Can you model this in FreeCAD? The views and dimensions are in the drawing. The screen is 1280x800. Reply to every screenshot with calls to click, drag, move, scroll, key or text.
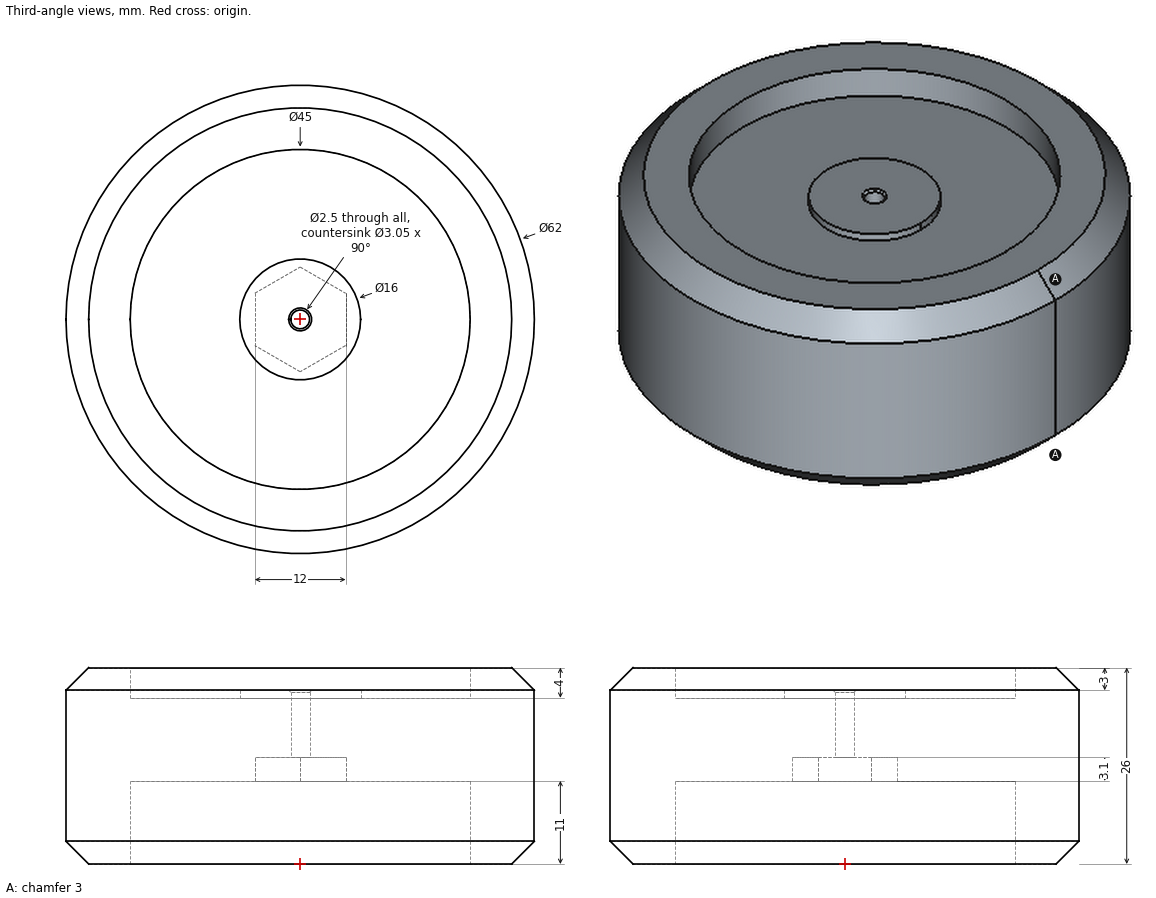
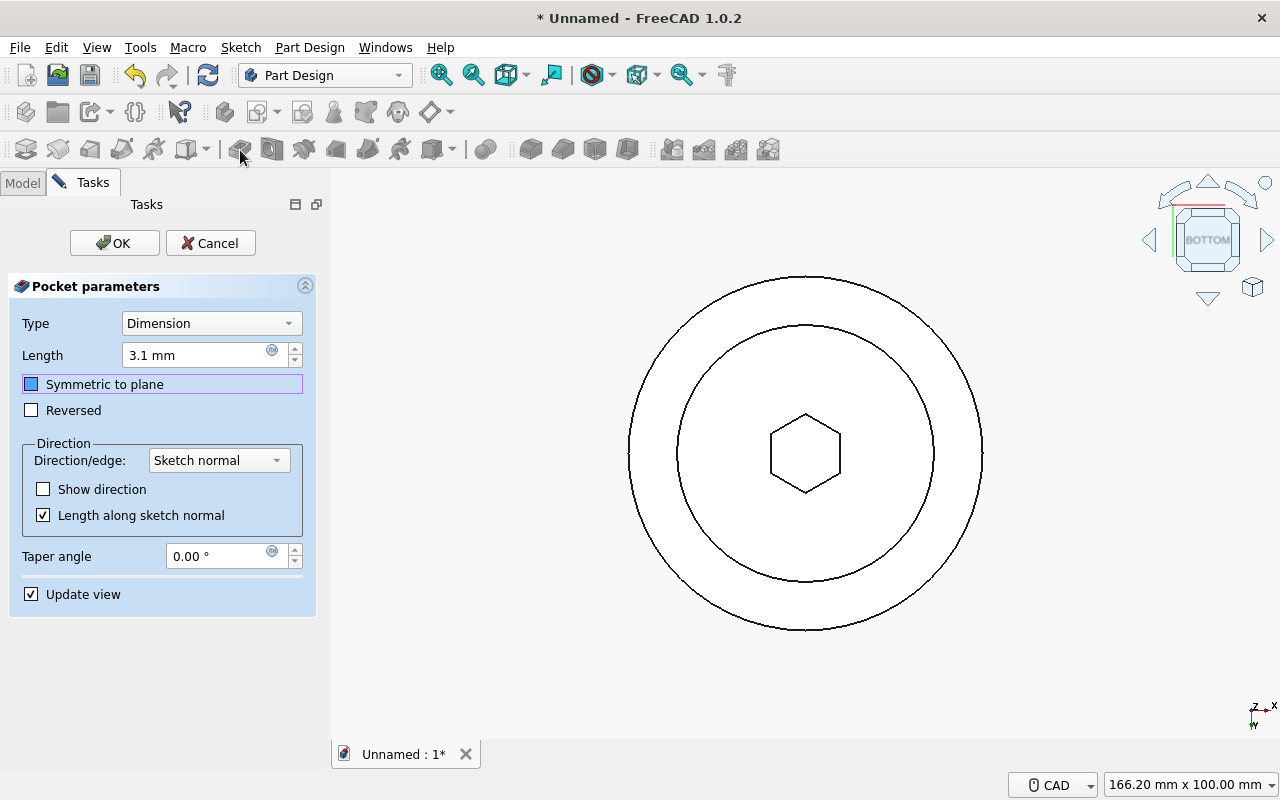
click(115, 243)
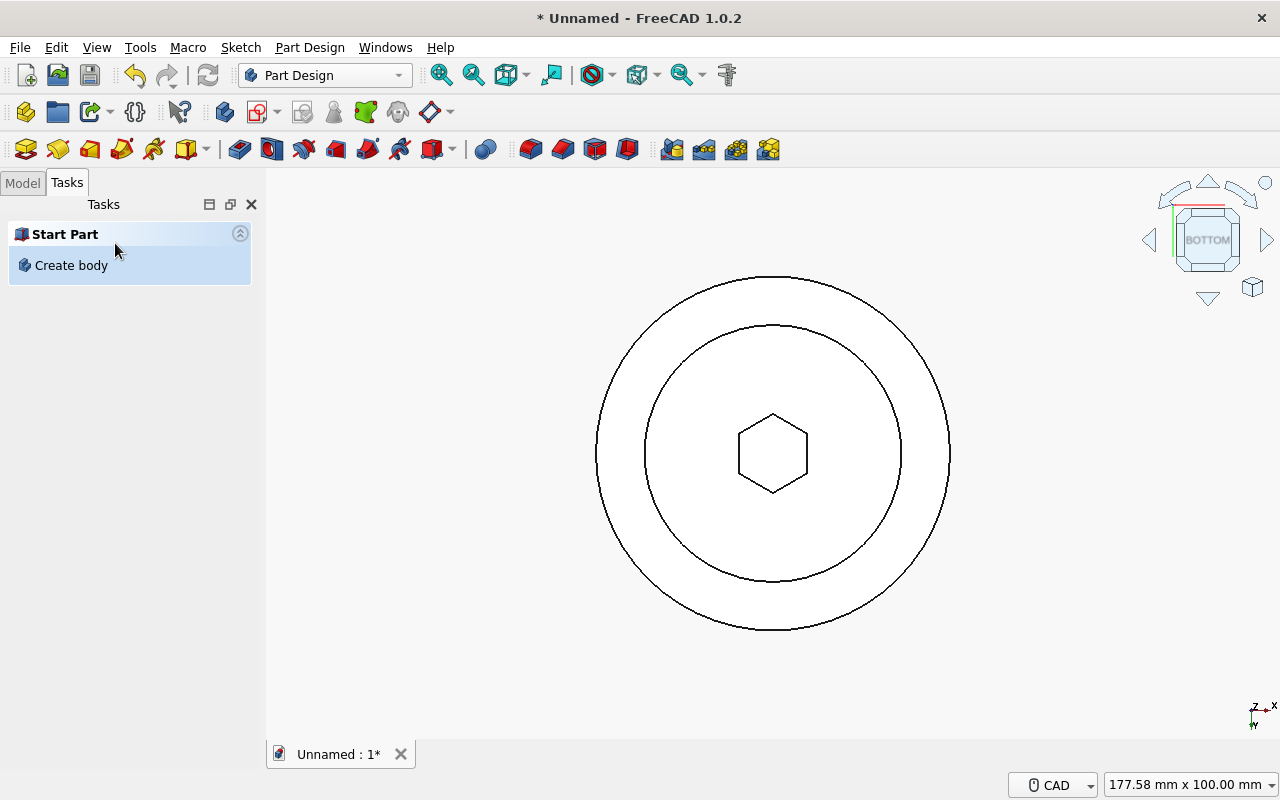
click(23, 182)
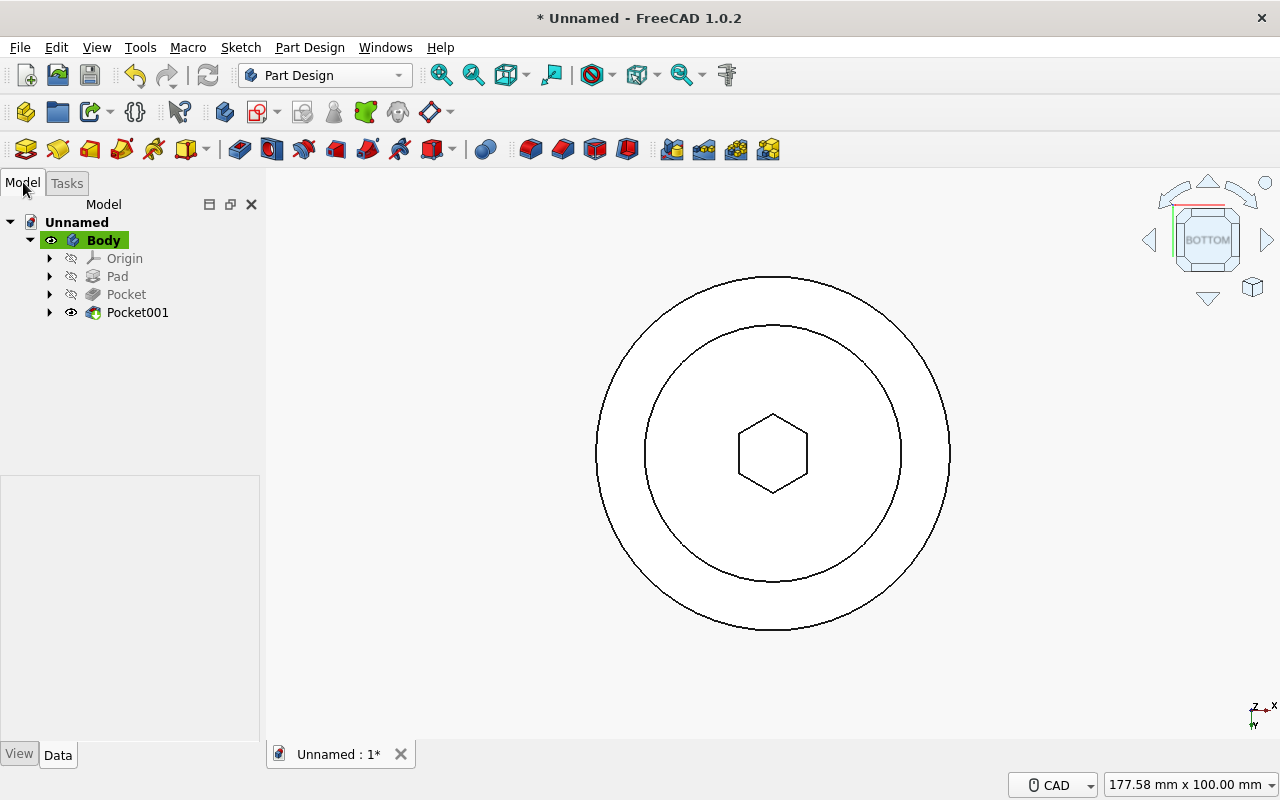
click(50, 258)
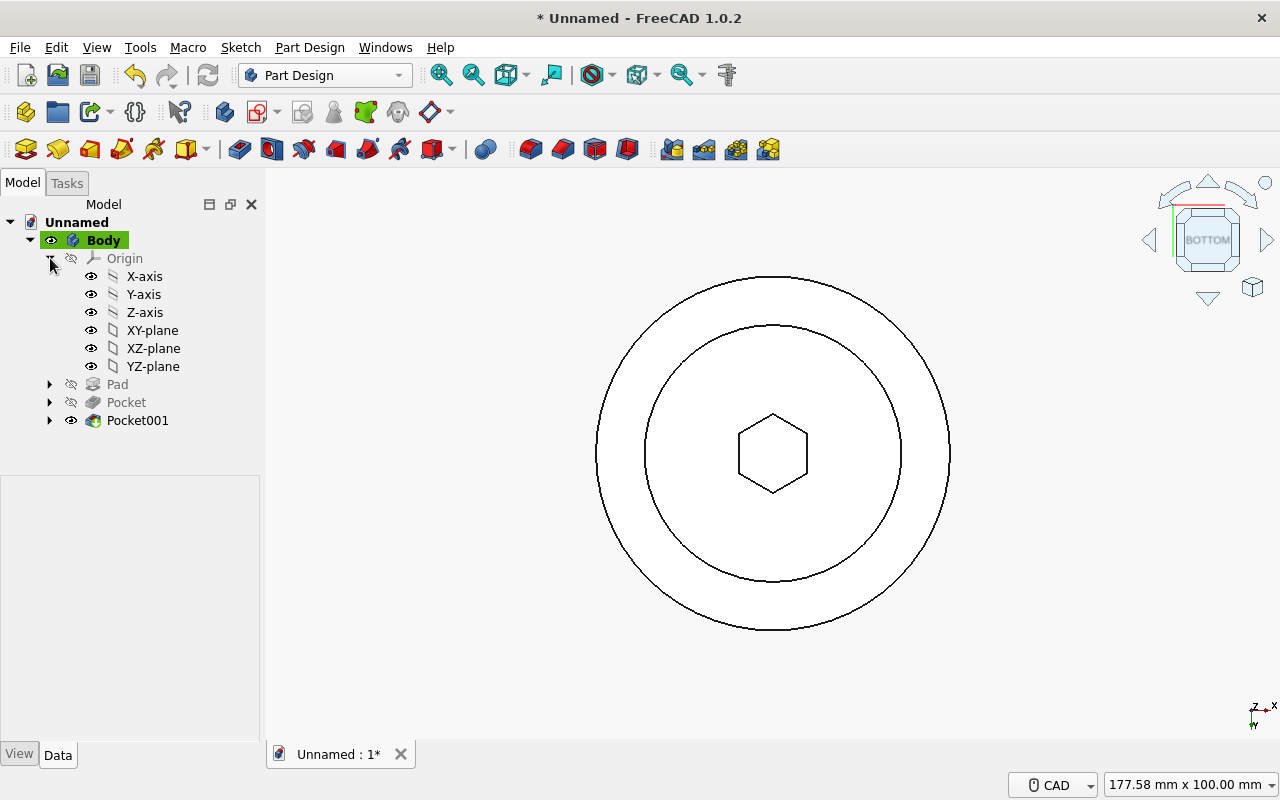
click(136, 330)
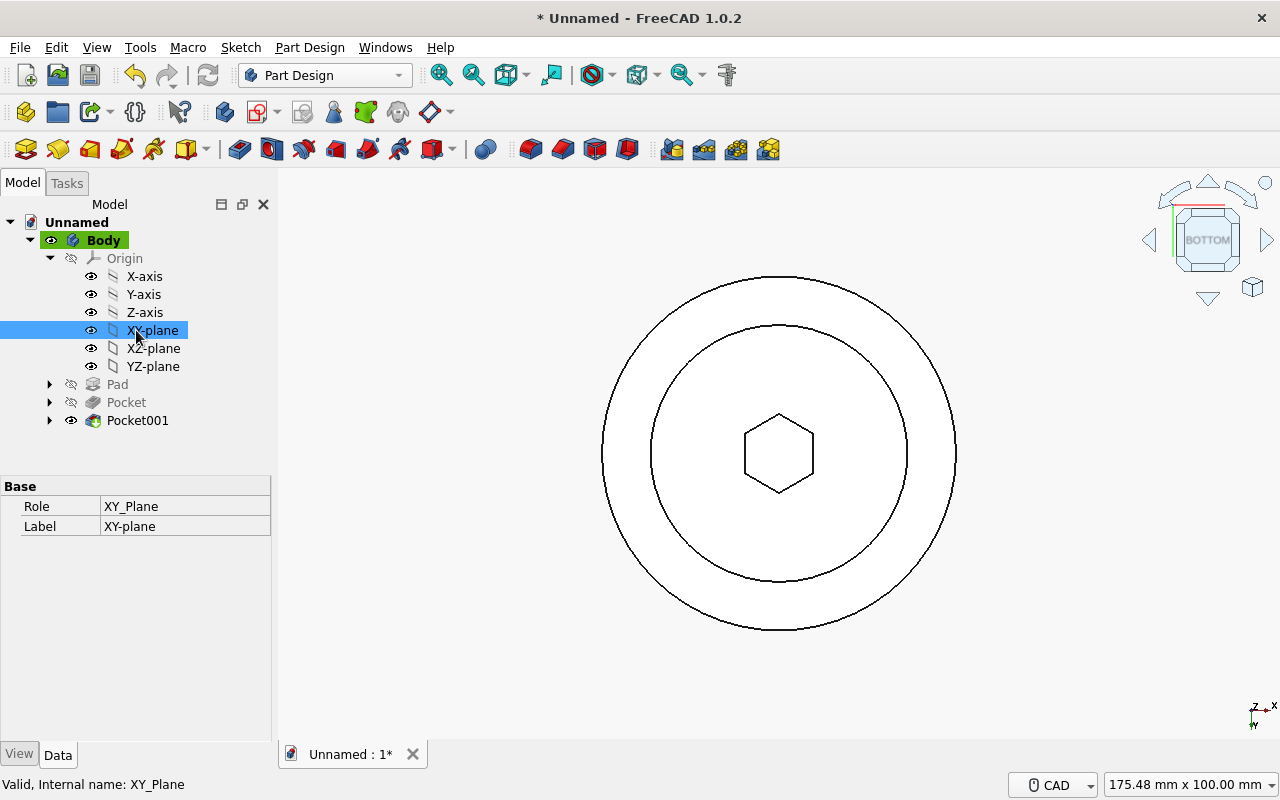
click(430, 112)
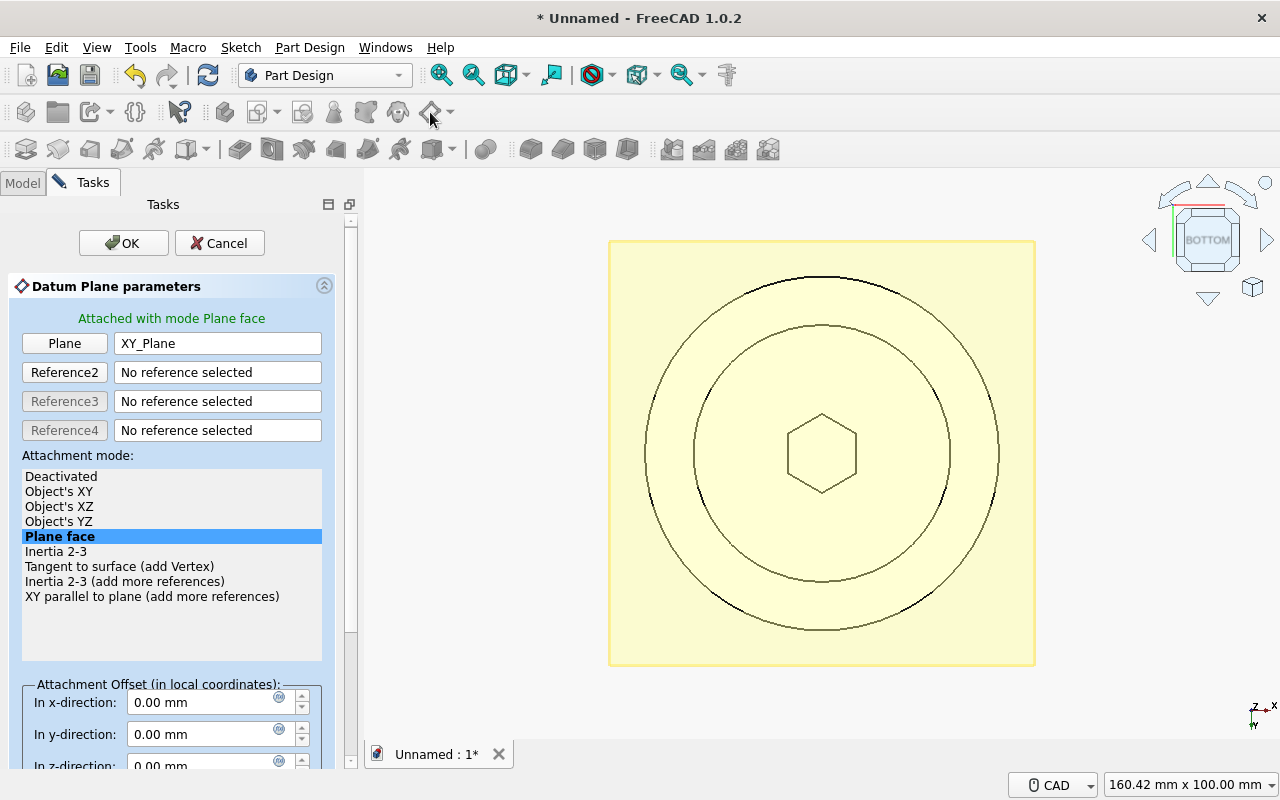
scroll(351, 491, down, 2)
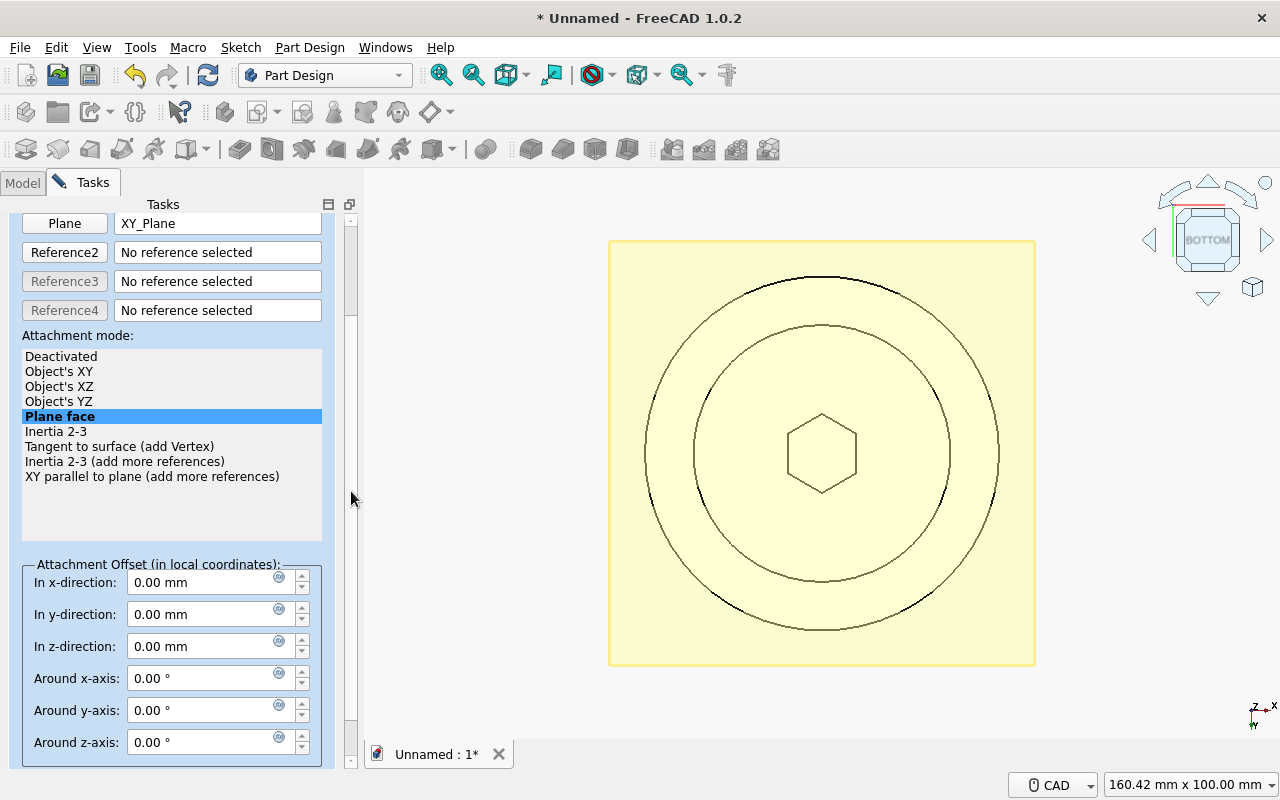
triple_click(210, 646)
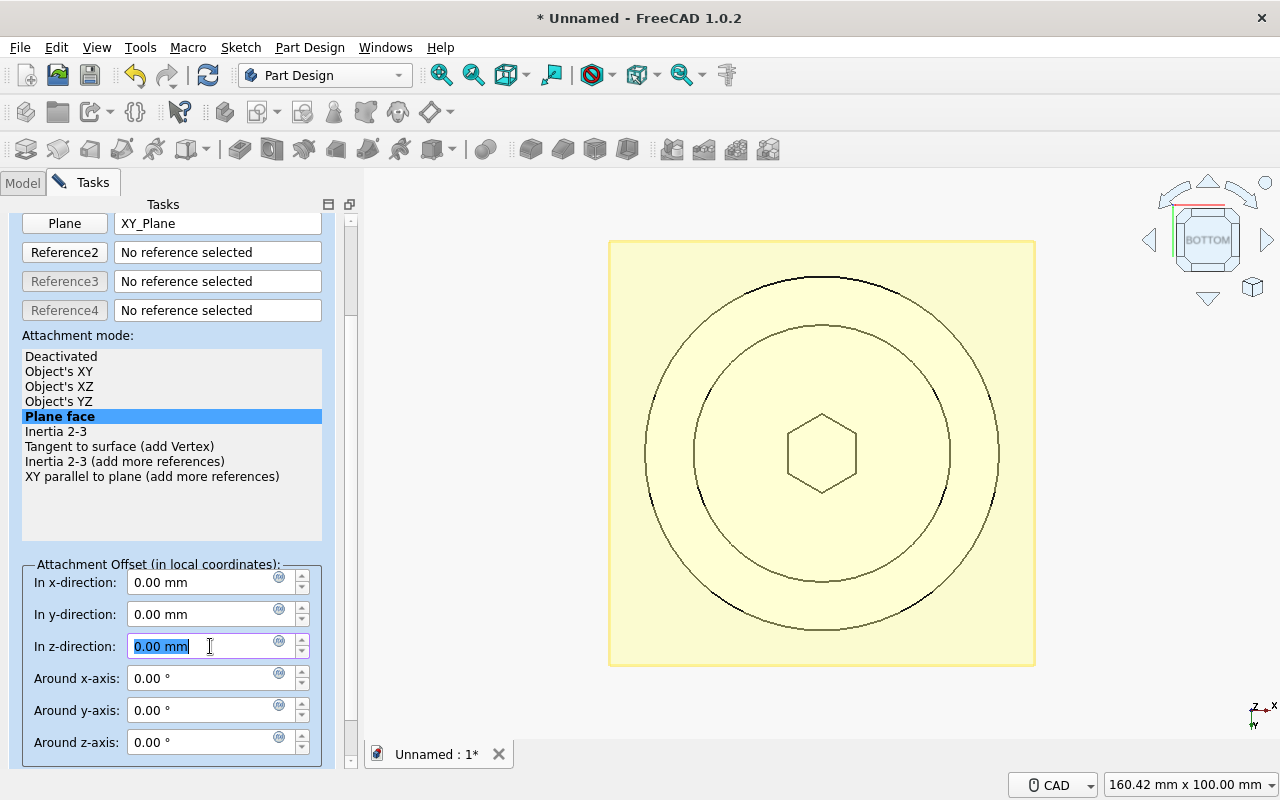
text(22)
key(Tab)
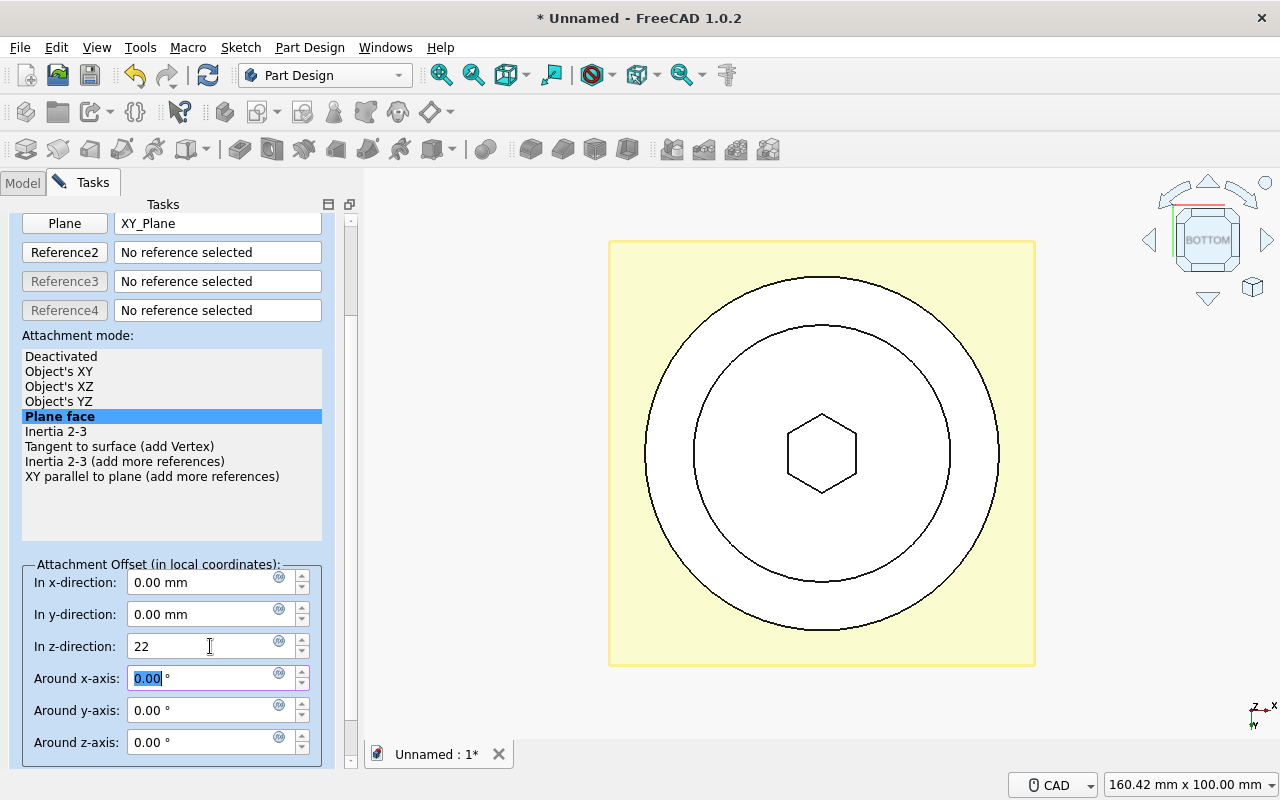
scroll(351, 491, up, 3)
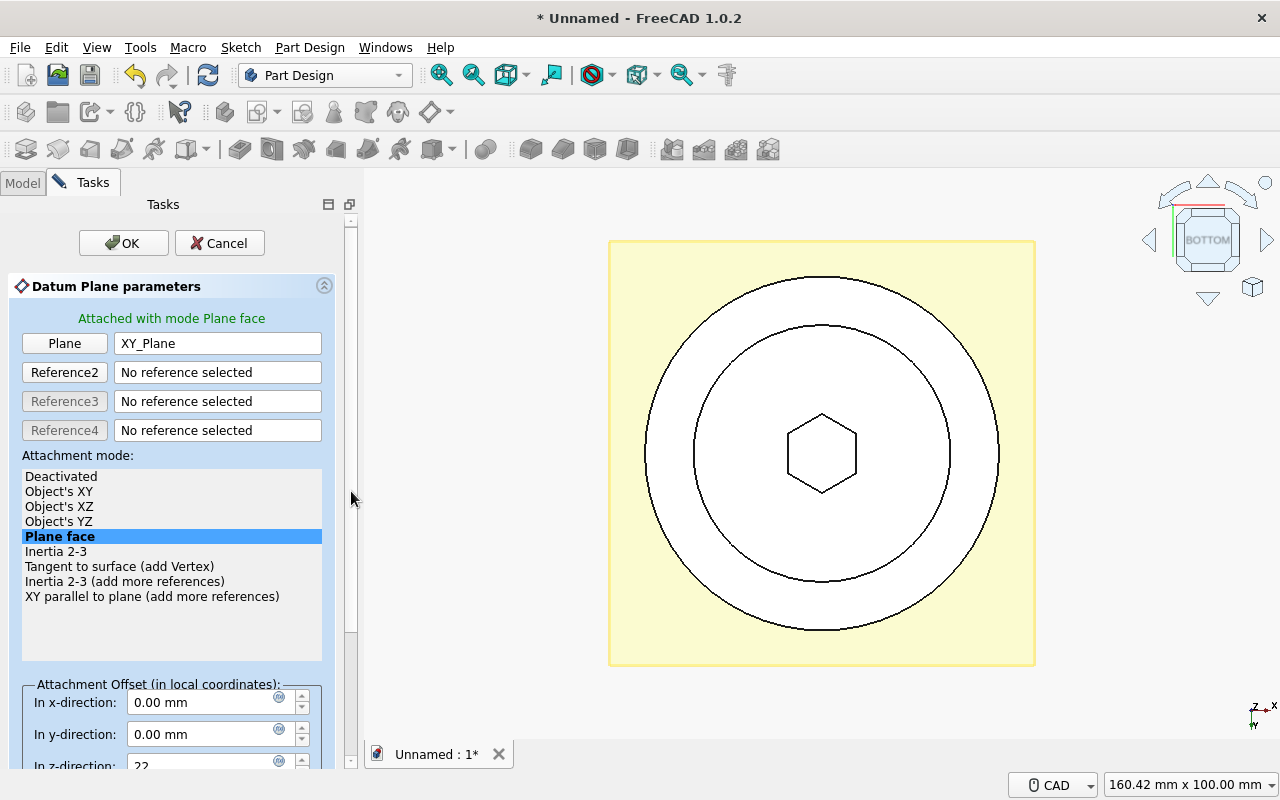
click(124, 243)